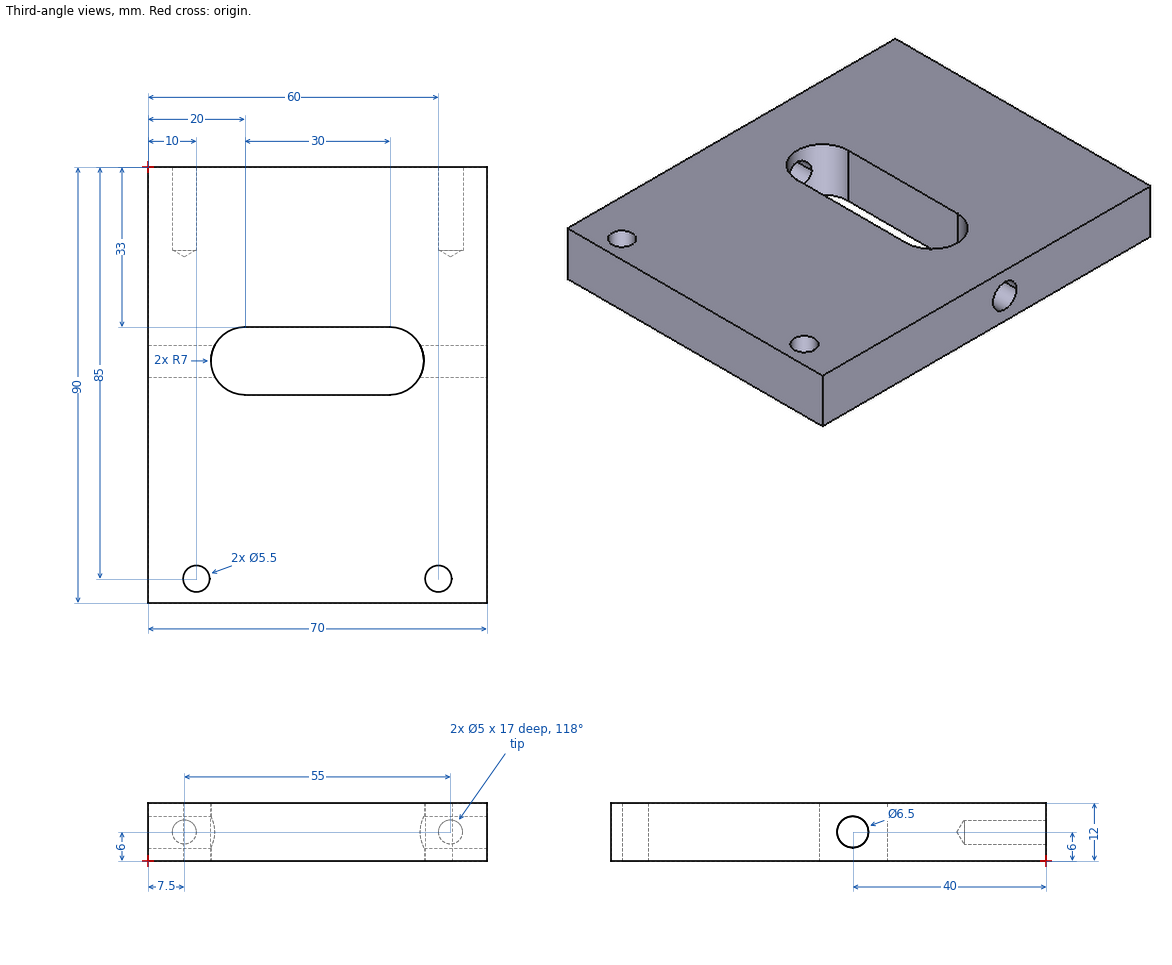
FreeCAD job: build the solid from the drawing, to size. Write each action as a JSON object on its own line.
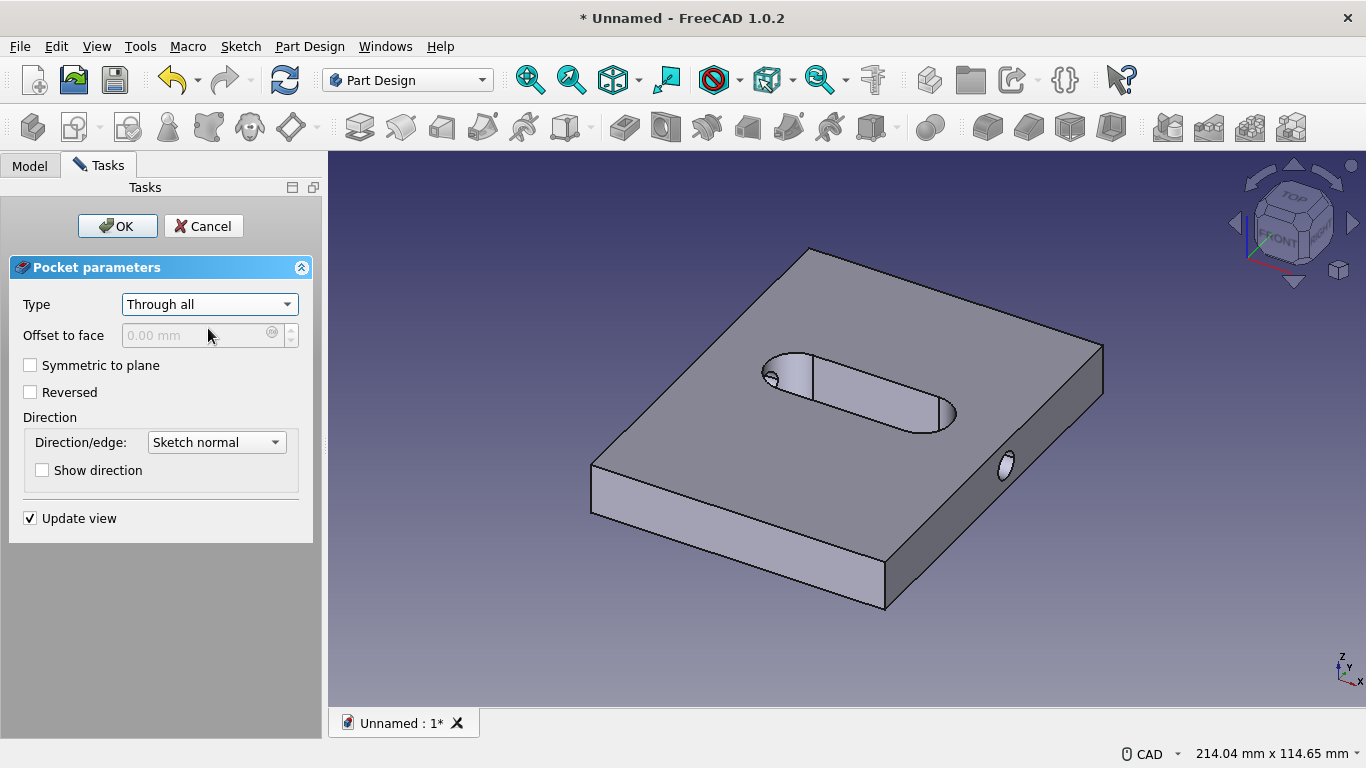
{"action": "left_click", "coordinate": [118, 226]}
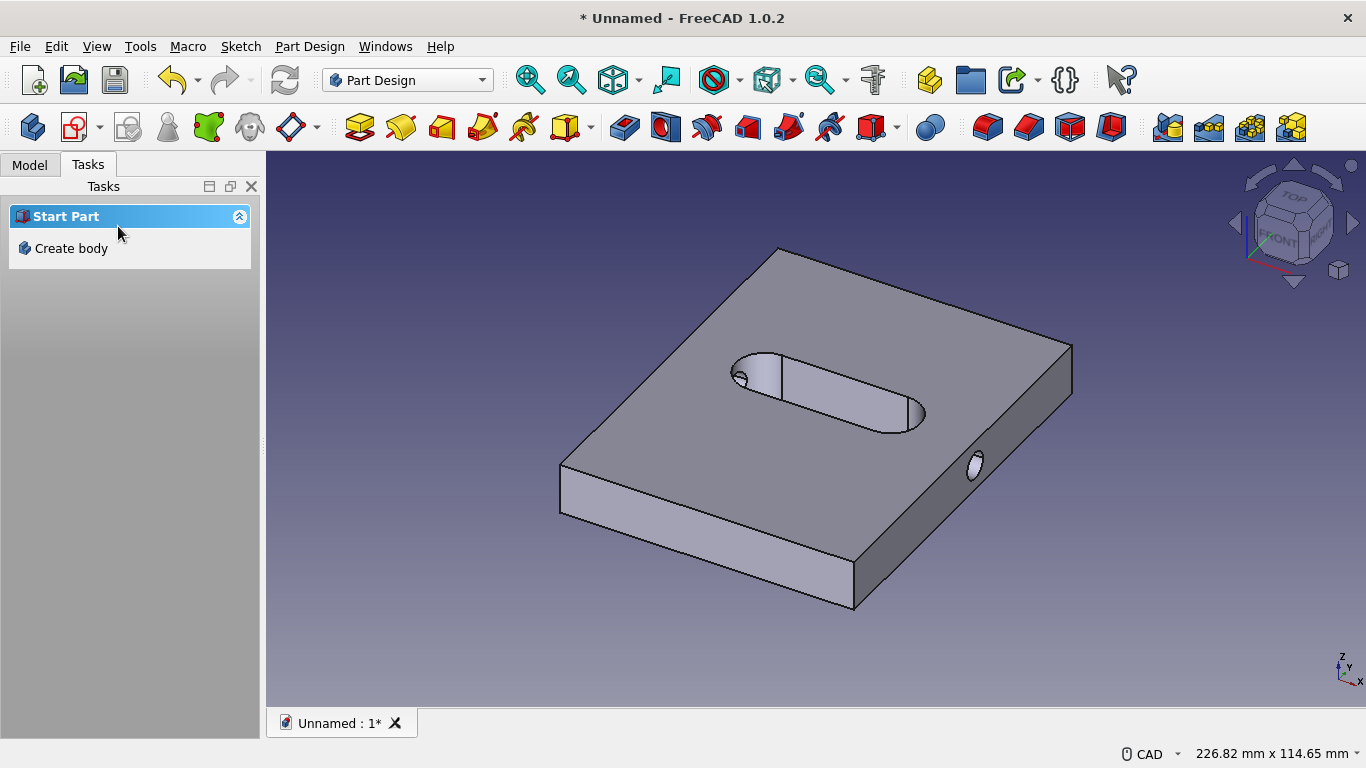
{"action": "left_click", "coordinate": [74, 128]}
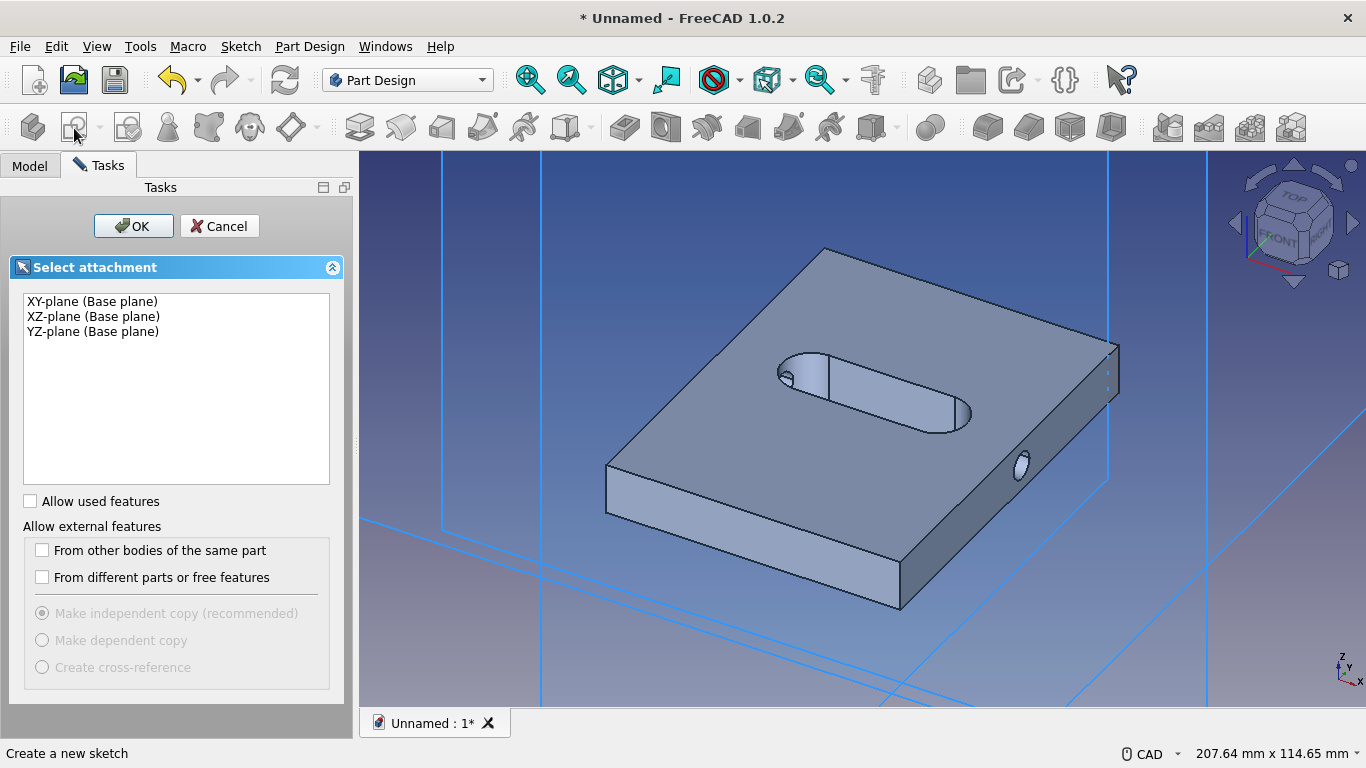
{"action": "left_click", "coordinate": [84, 316]}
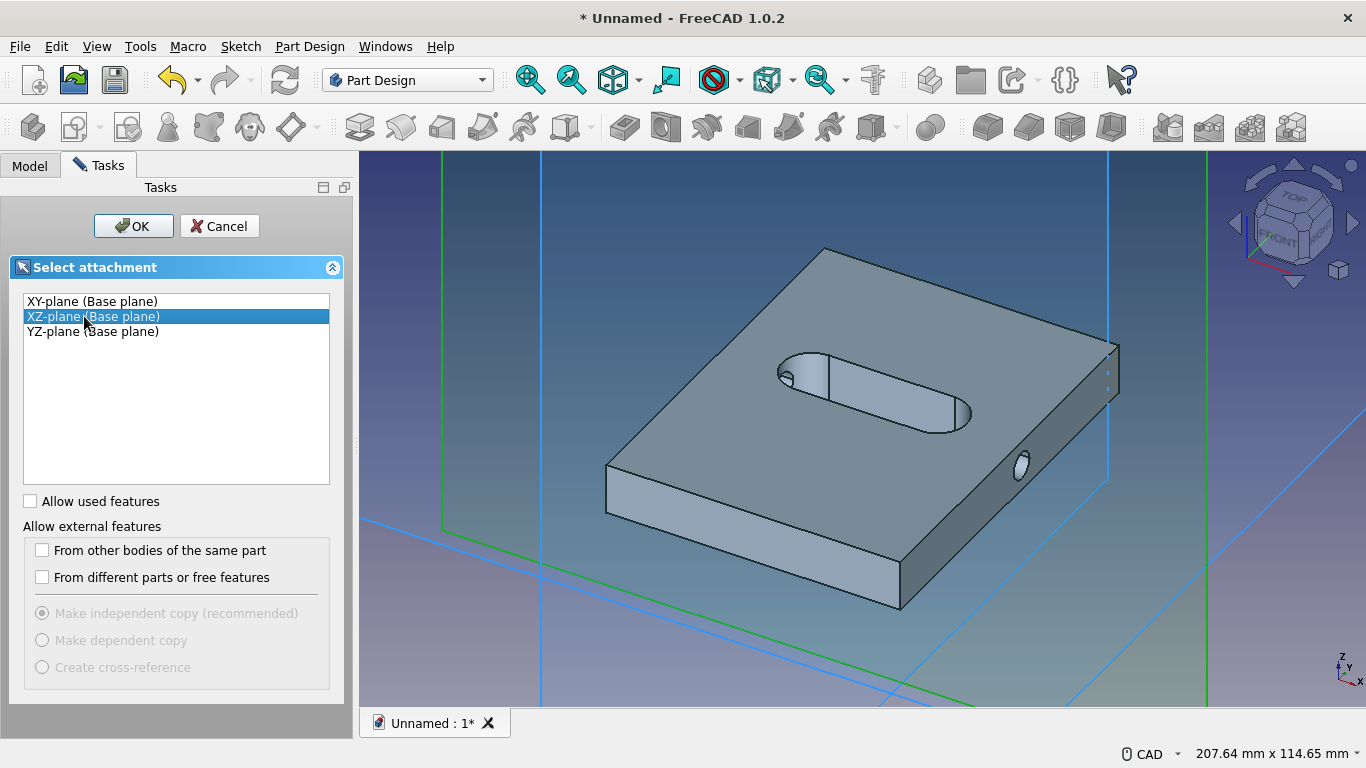
{"action": "left_click", "coordinate": [134, 226]}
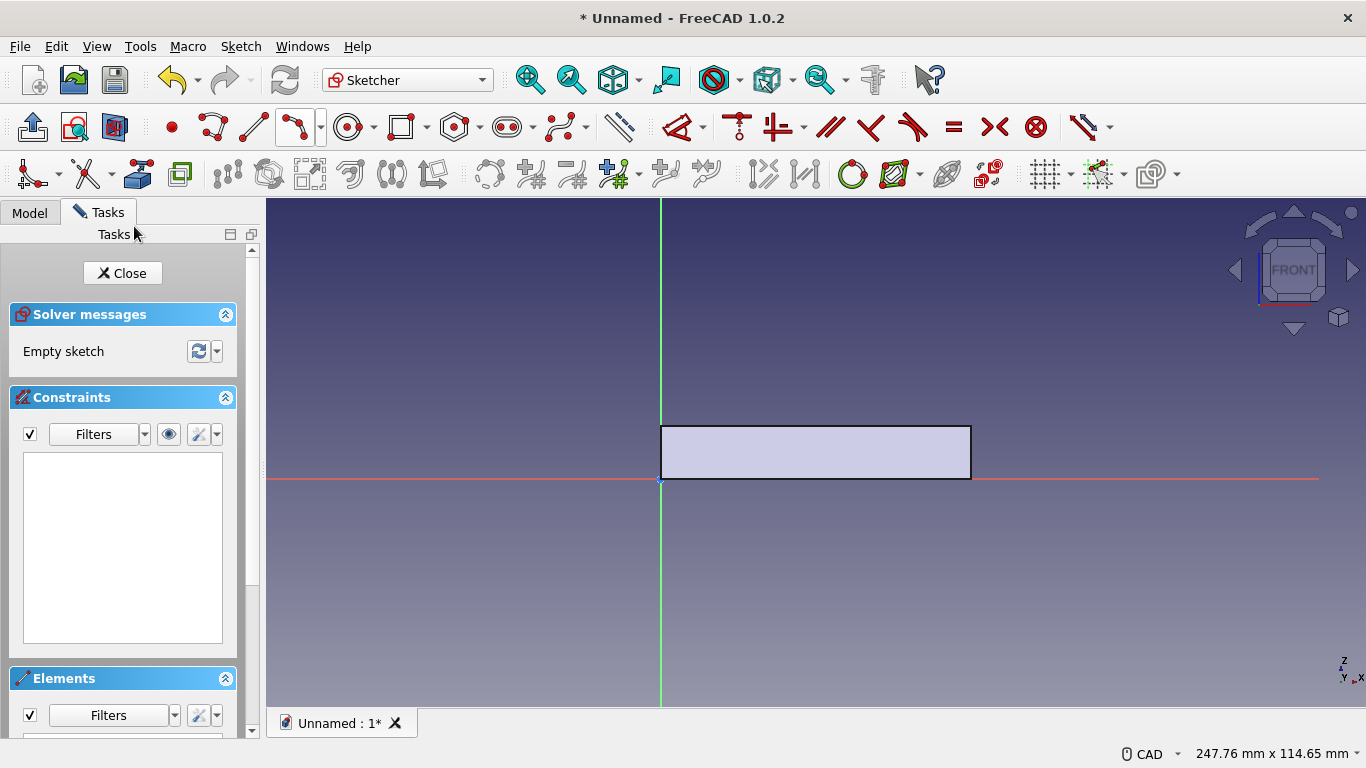
{"action": "left_click", "coordinate": [115, 128]}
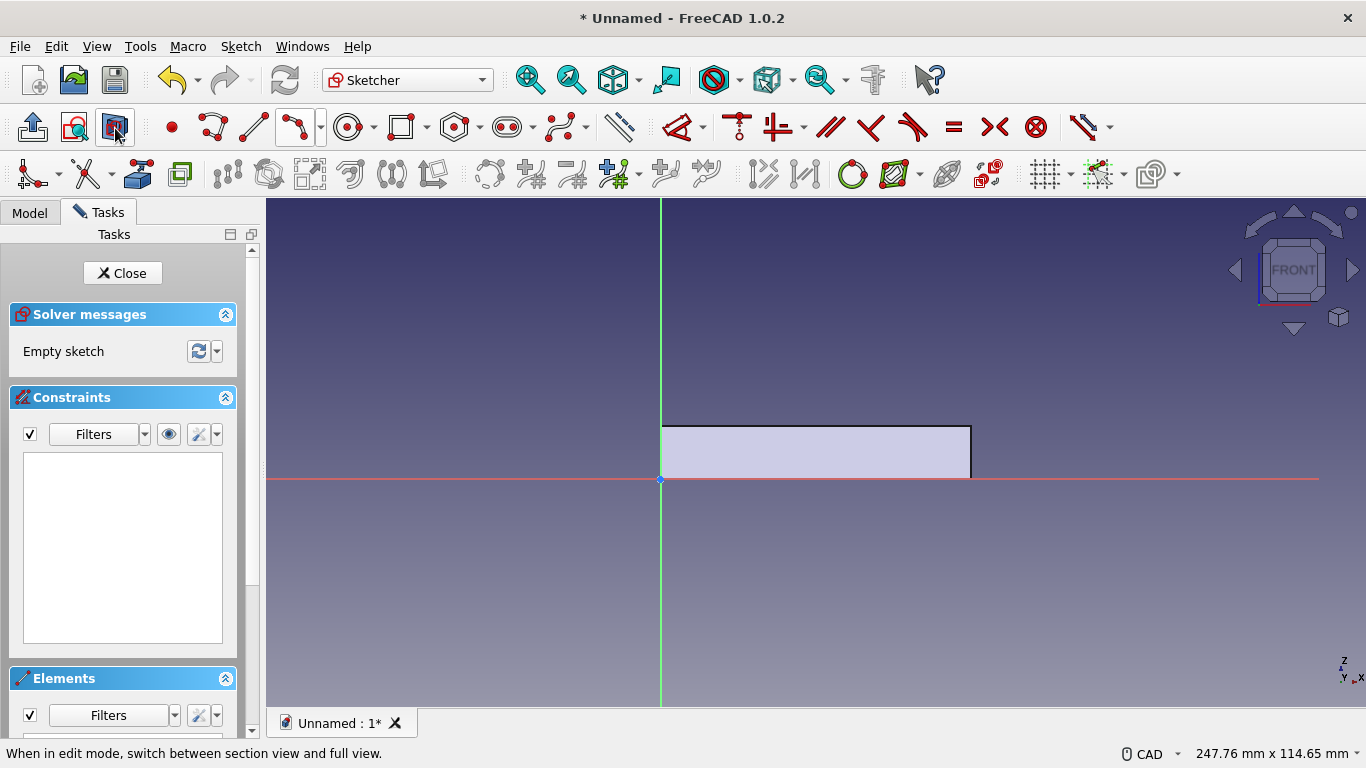
{"action": "scroll", "coordinate": [852, 467], "scroll_direction": "up", "scroll_amount": 4}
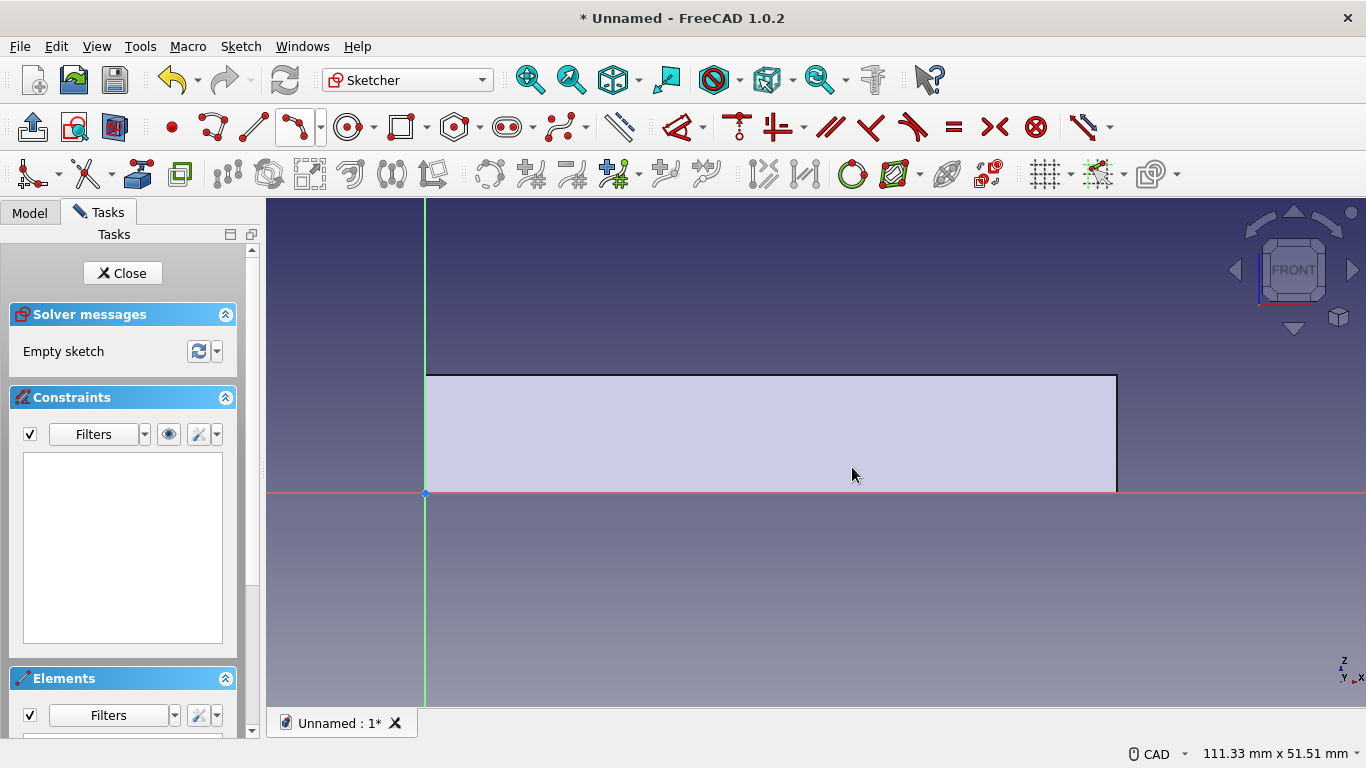
{"action": "left_click", "coordinate": [348, 128]}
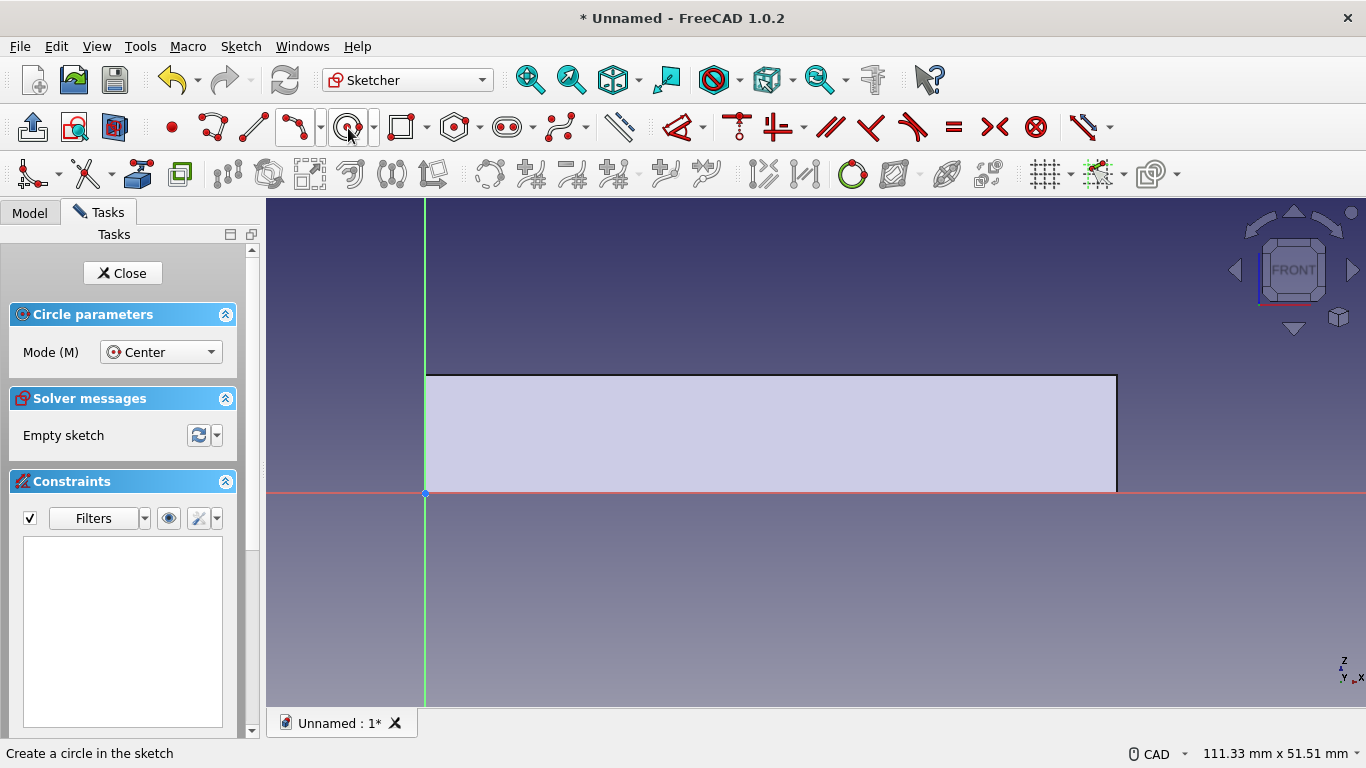
{"action": "left_click", "coordinate": [1043, 434]}
{"action": "left_click", "coordinate": [1060, 417]}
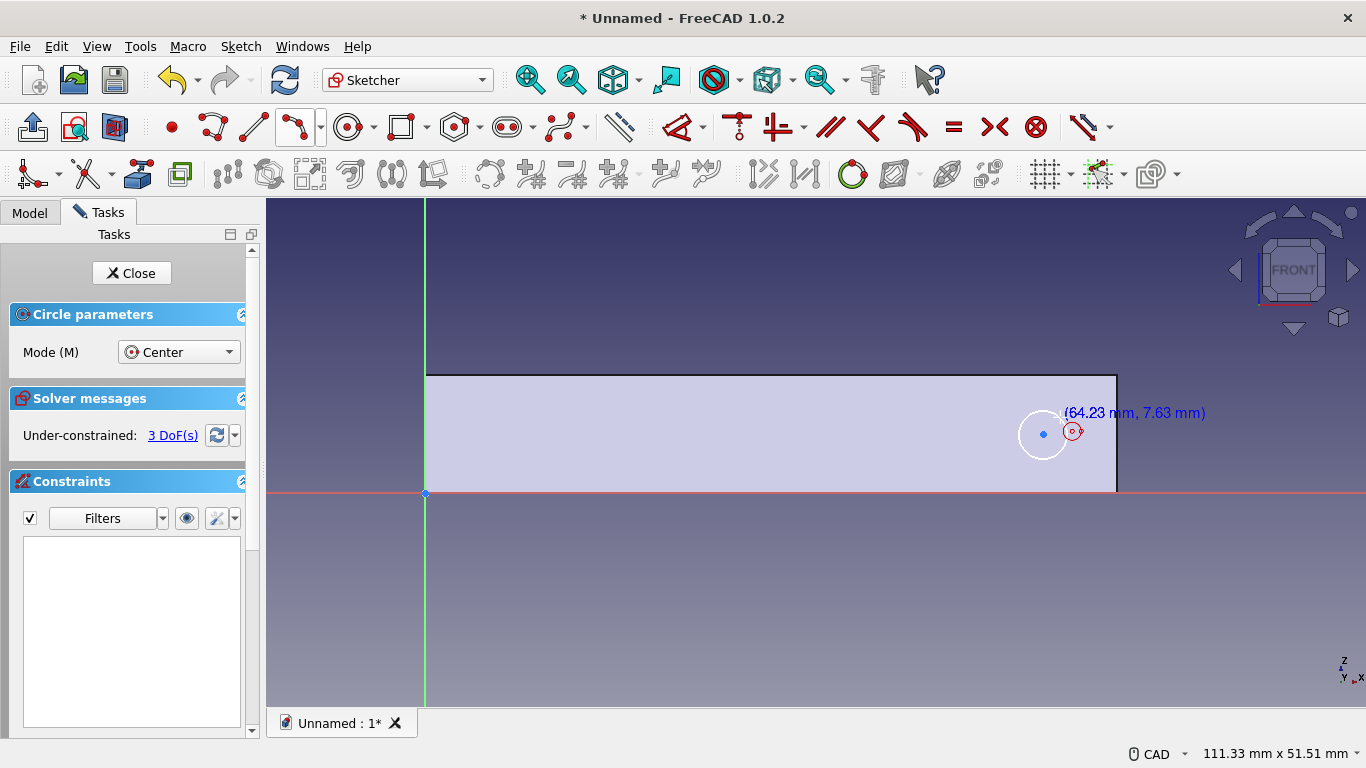
{"action": "left_click", "coordinate": [500, 434]}
{"action": "left_click", "coordinate": [517, 417]}
{"action": "key", "text": "Escape"}